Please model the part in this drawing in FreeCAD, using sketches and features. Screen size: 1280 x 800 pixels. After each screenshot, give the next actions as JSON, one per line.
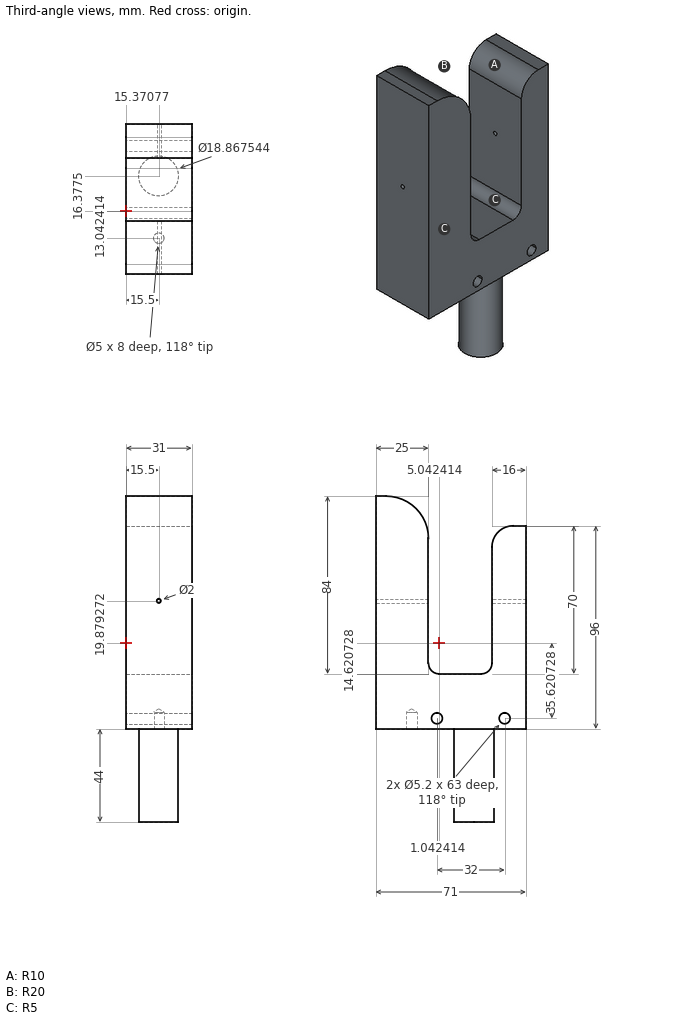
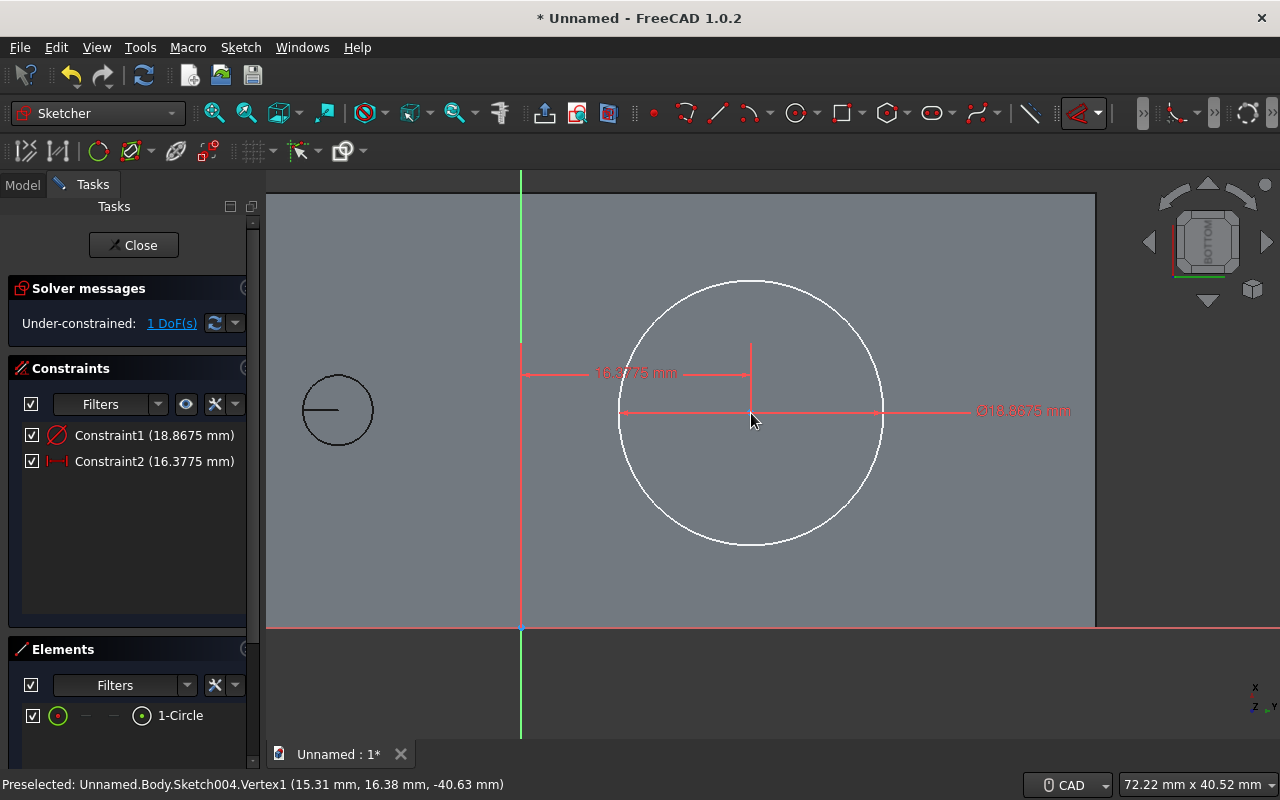
{"action": "left_click", "coordinate": [751, 413]}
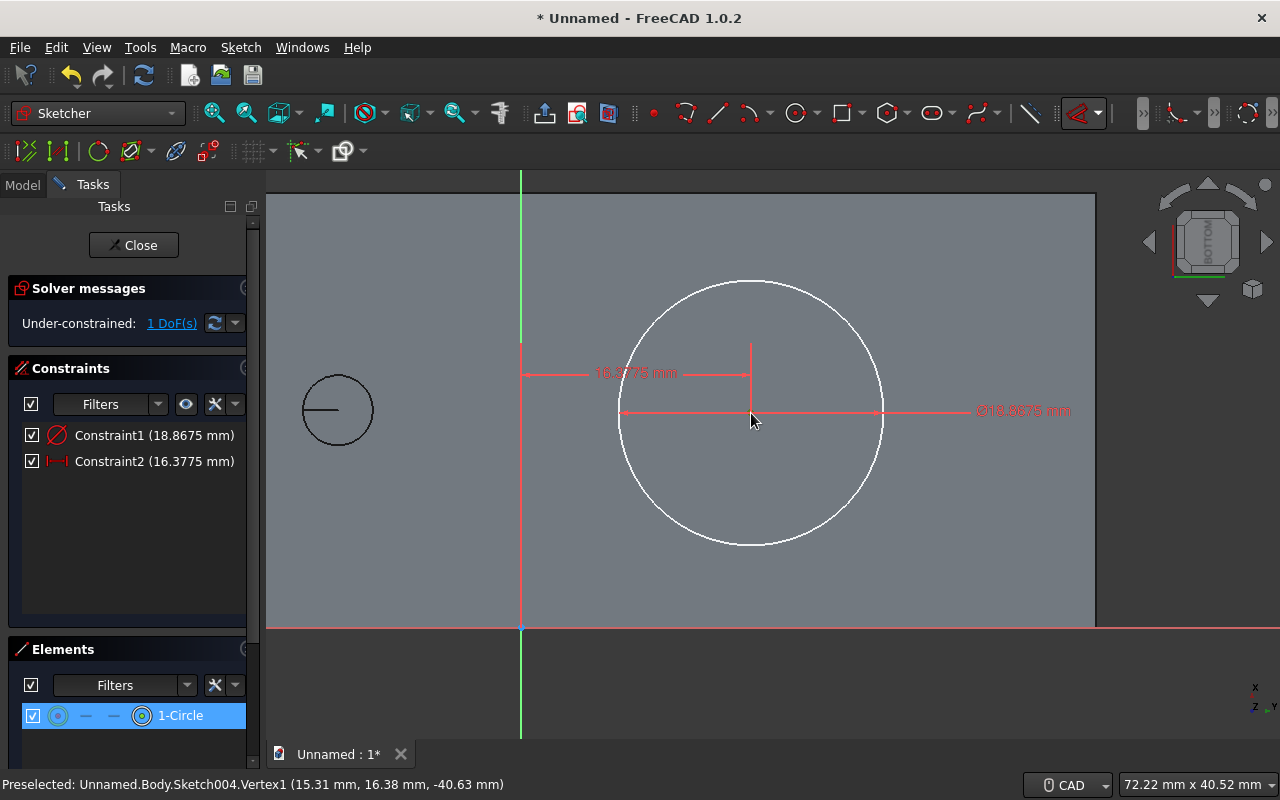
{"action": "left_click", "coordinate": [1100, 114]}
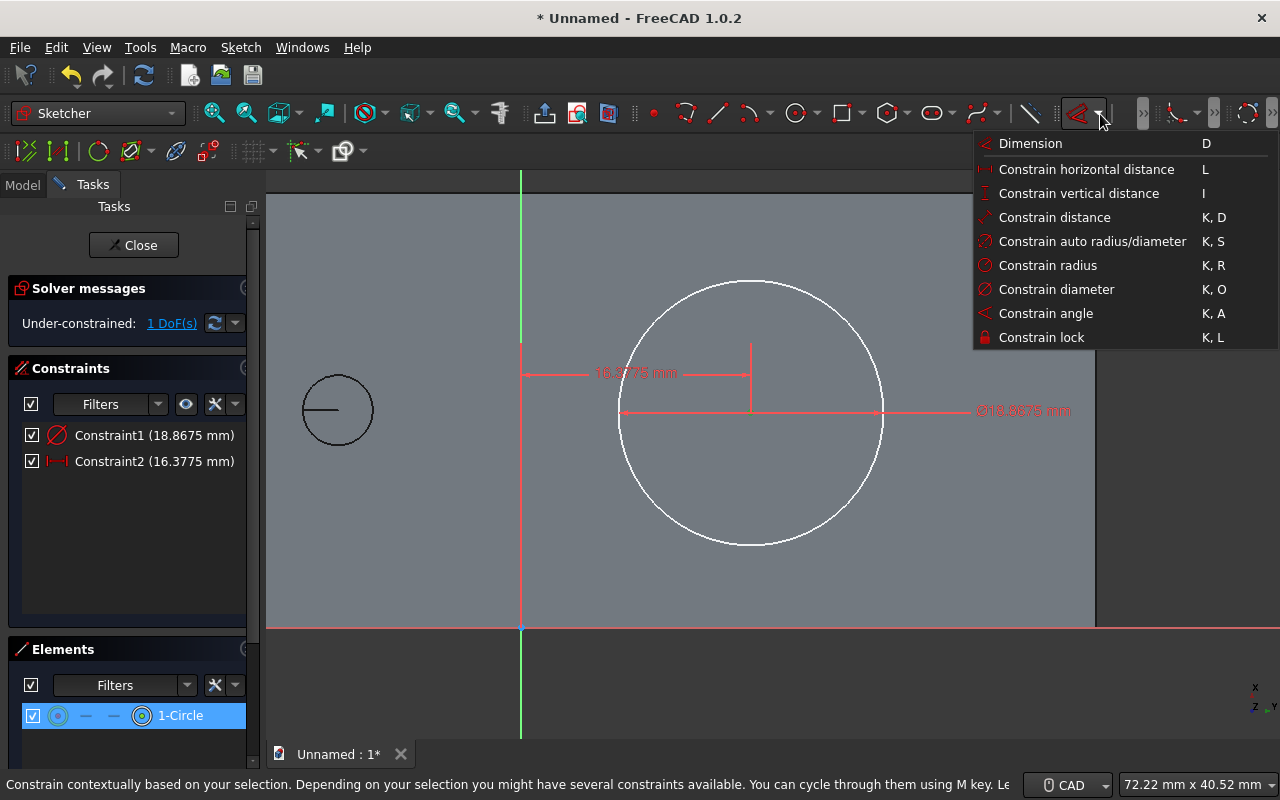
{"action": "left_click", "coordinate": [1126, 193]}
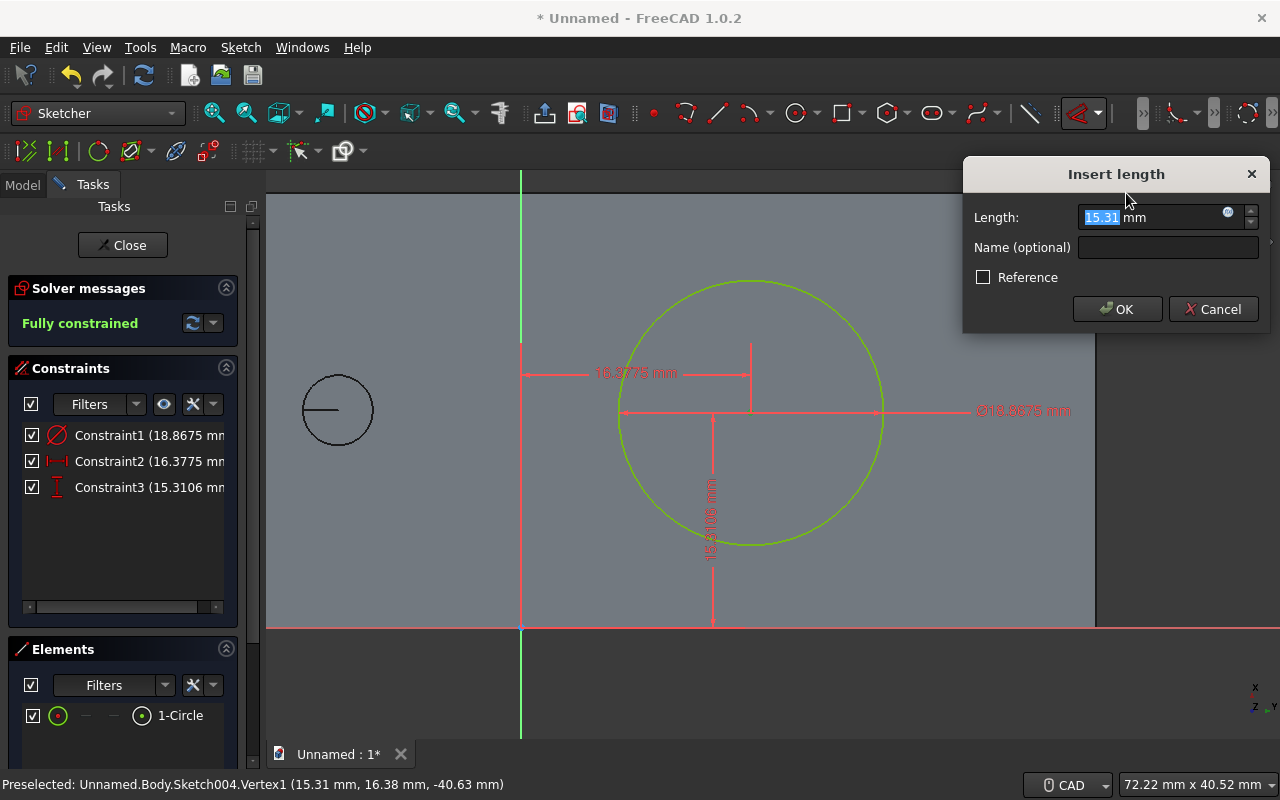
{"action": "type", "text": "15.37077"}
{"action": "key", "text": "Return"}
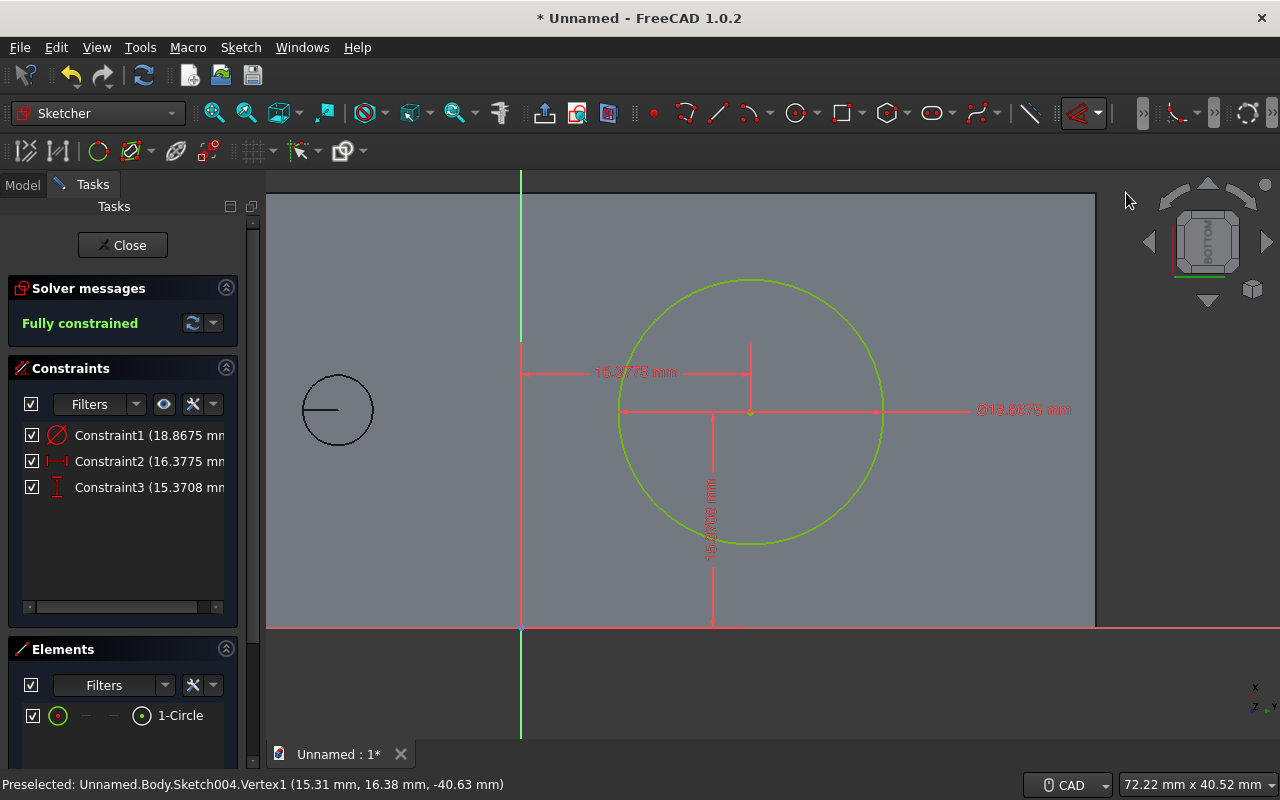
{"action": "left_click", "coordinate": [123, 245]}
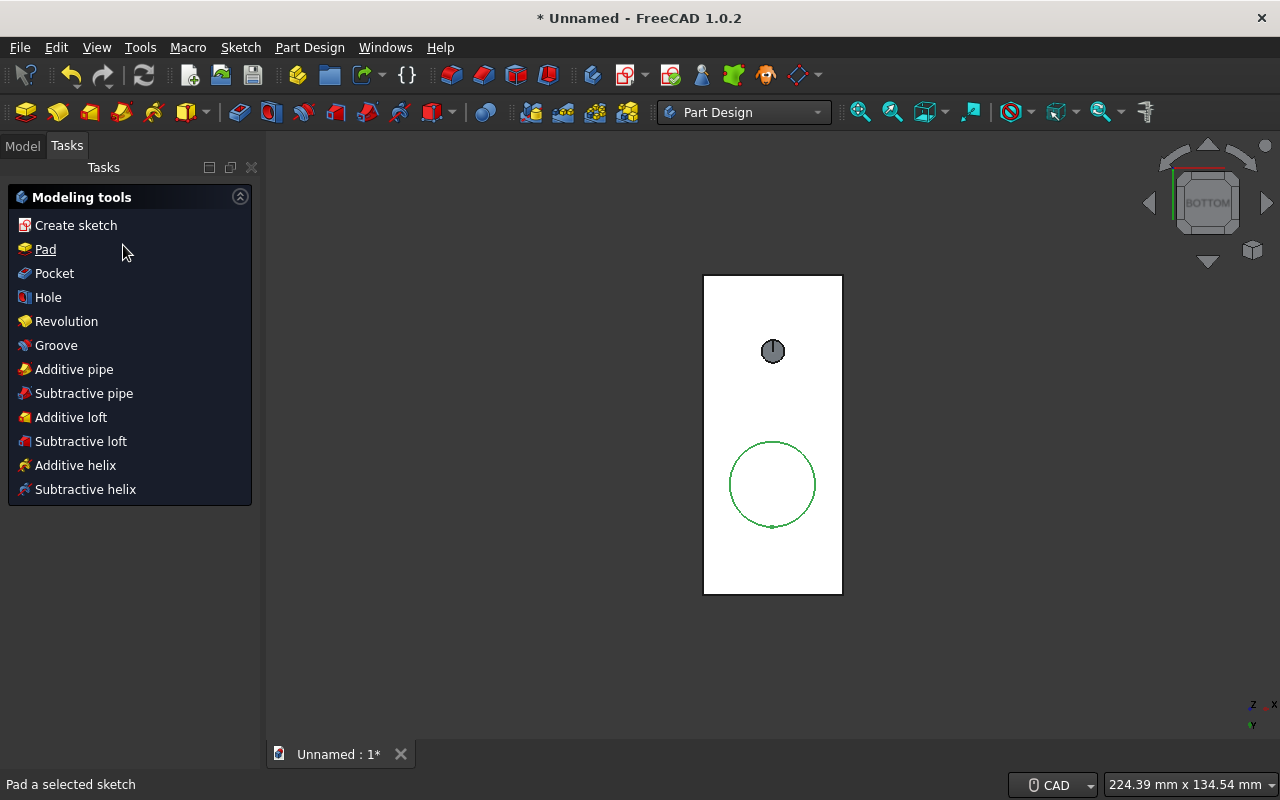
{"action": "left_click", "coordinate": [26, 112]}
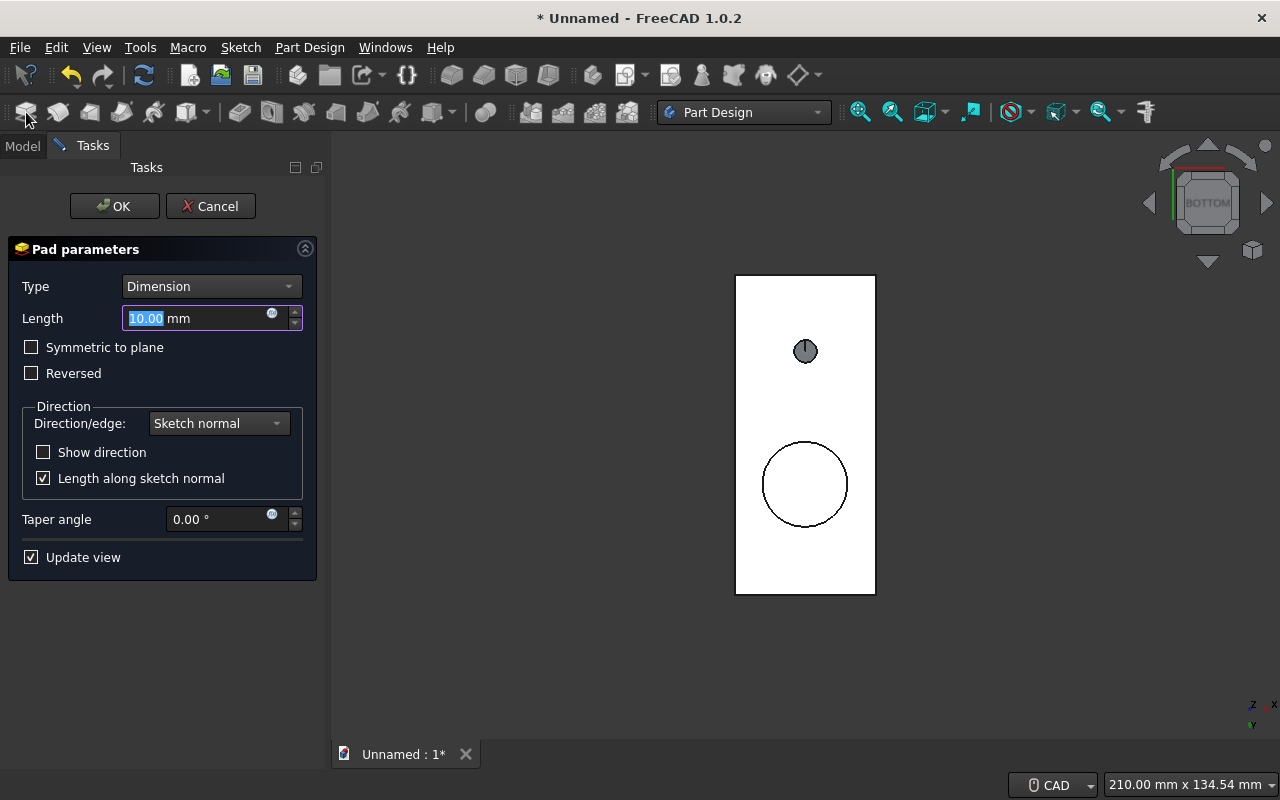
{"action": "type", "text": "44"}
{"action": "key", "text": "Tab"}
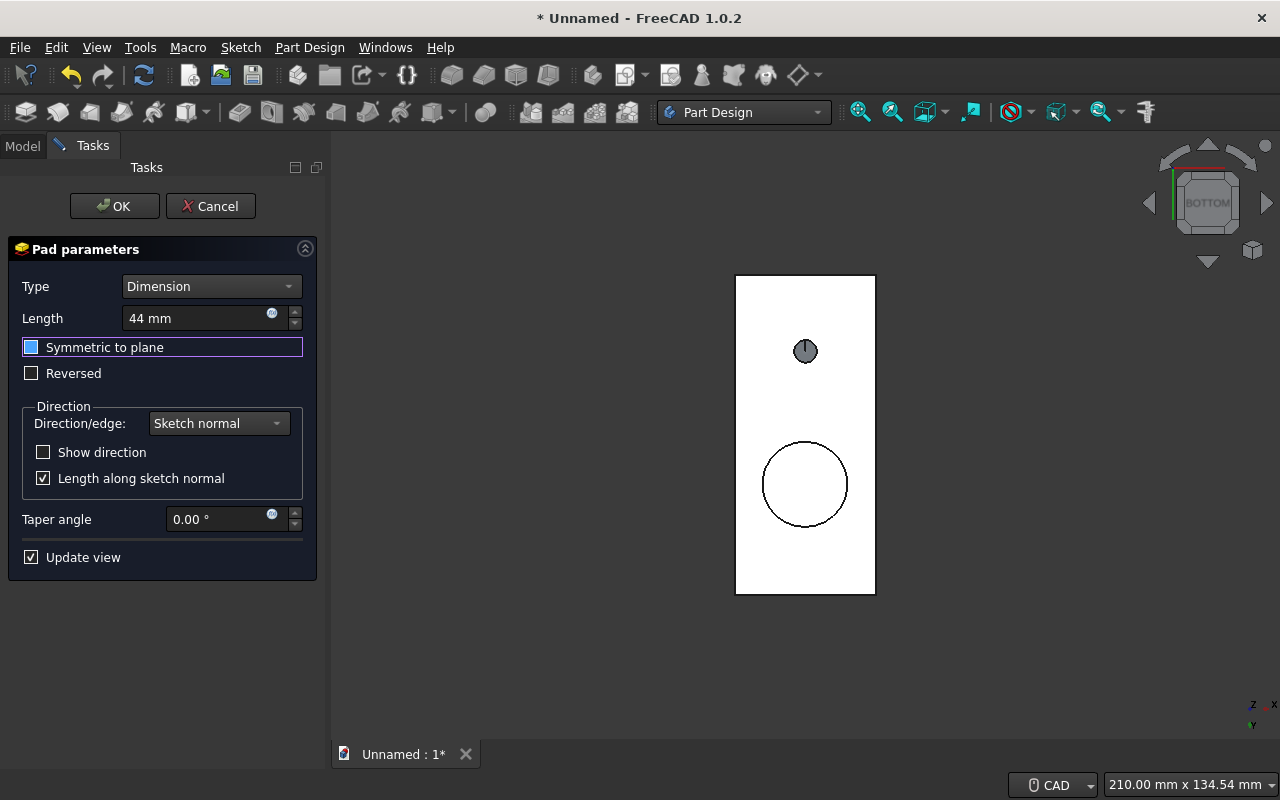
{"action": "left_click", "coordinate": [115, 206]}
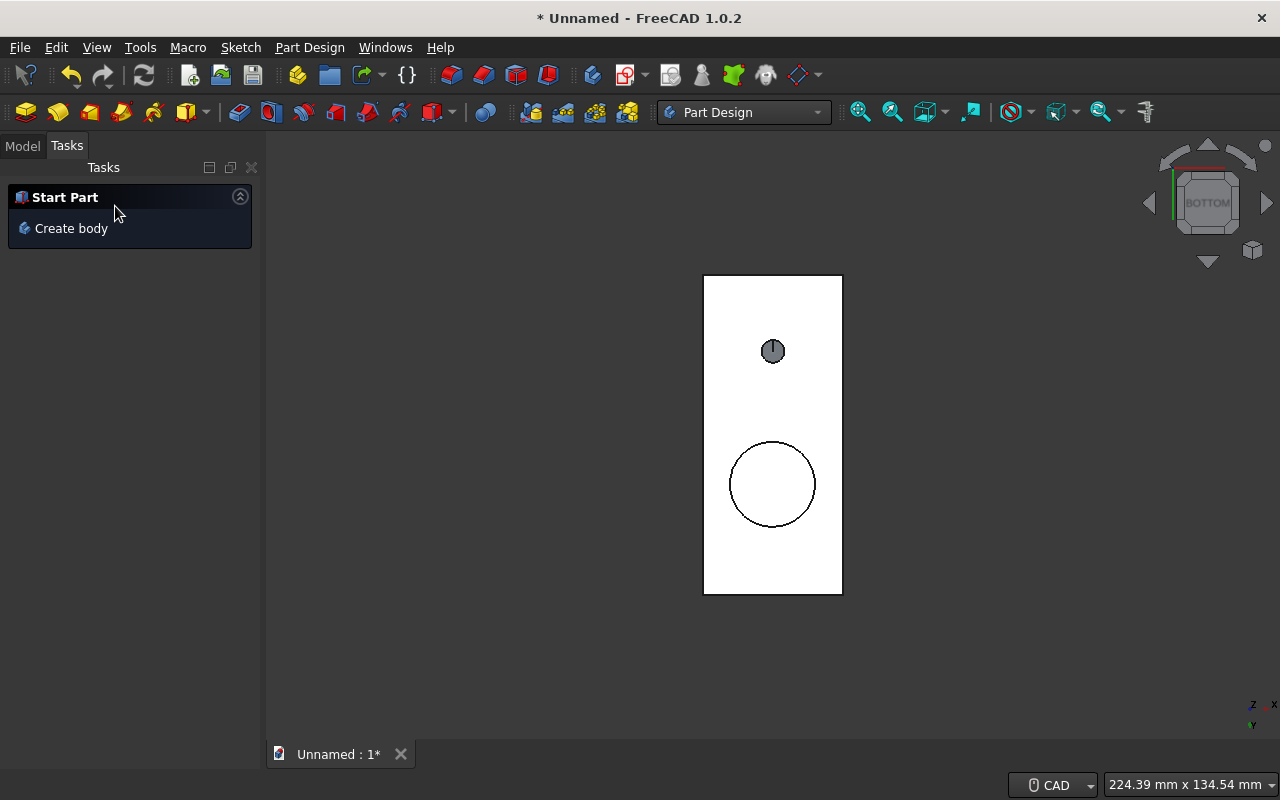
{"action": "key", "text": "0"}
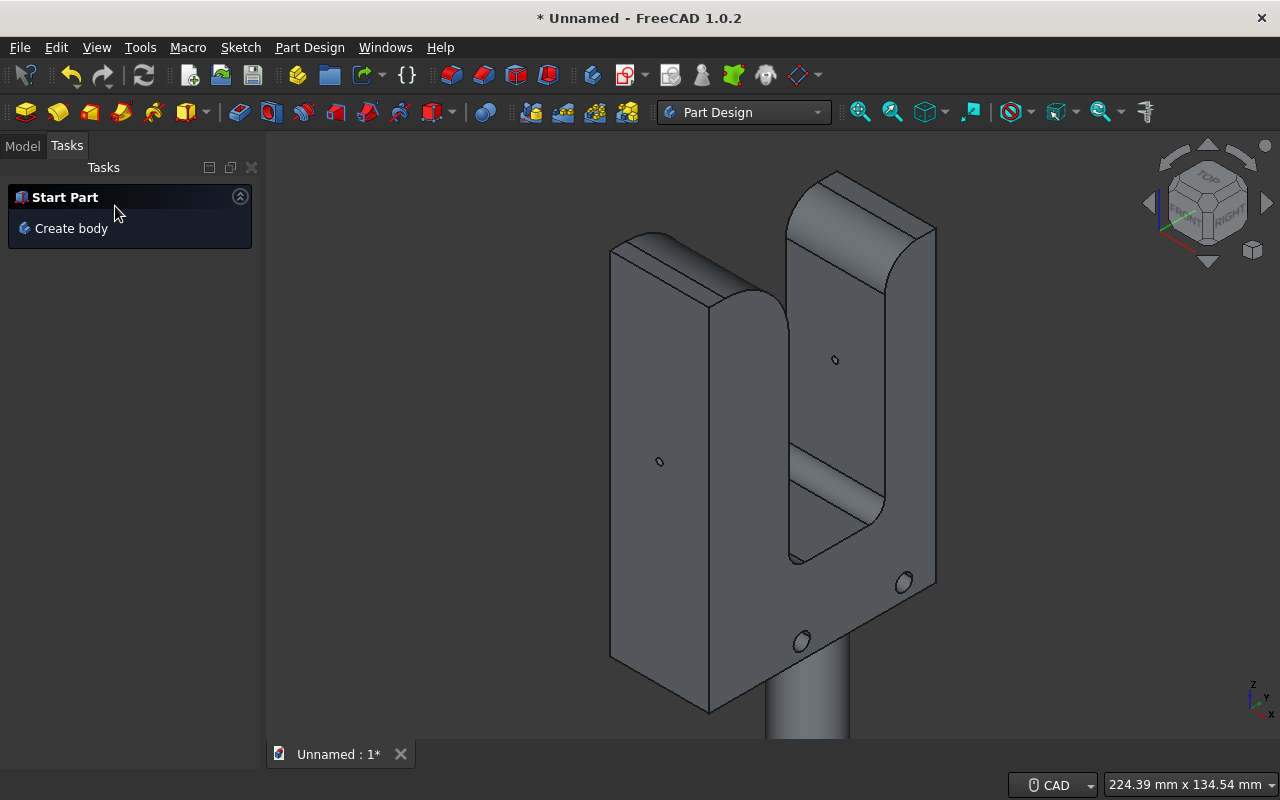
{"action": "key", "text": "v f"}